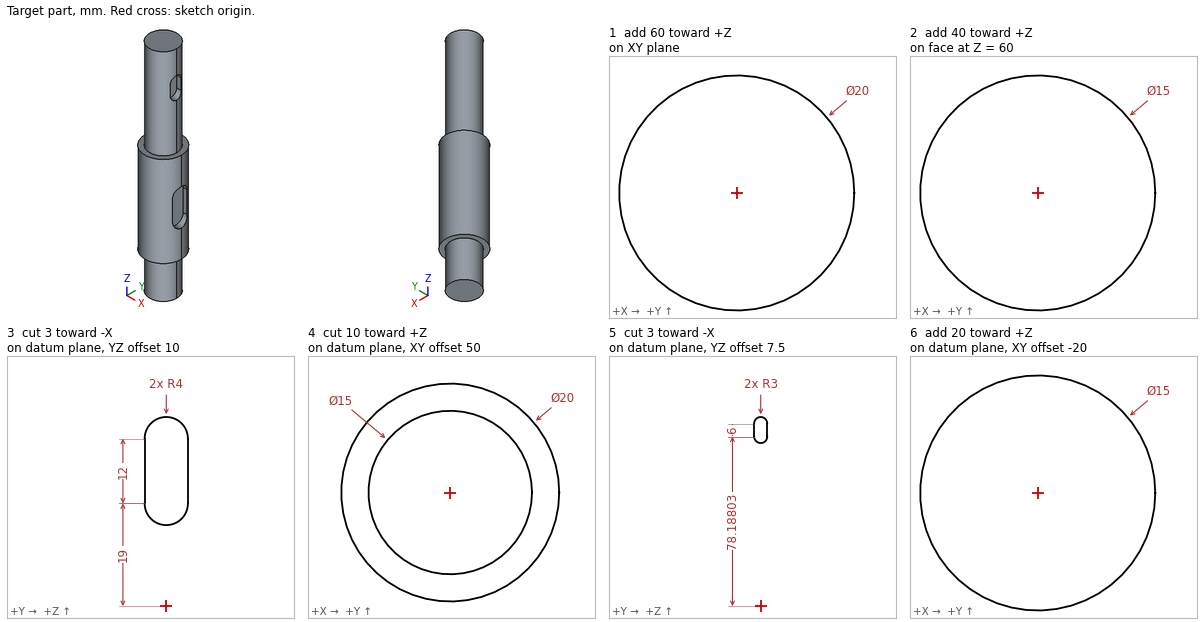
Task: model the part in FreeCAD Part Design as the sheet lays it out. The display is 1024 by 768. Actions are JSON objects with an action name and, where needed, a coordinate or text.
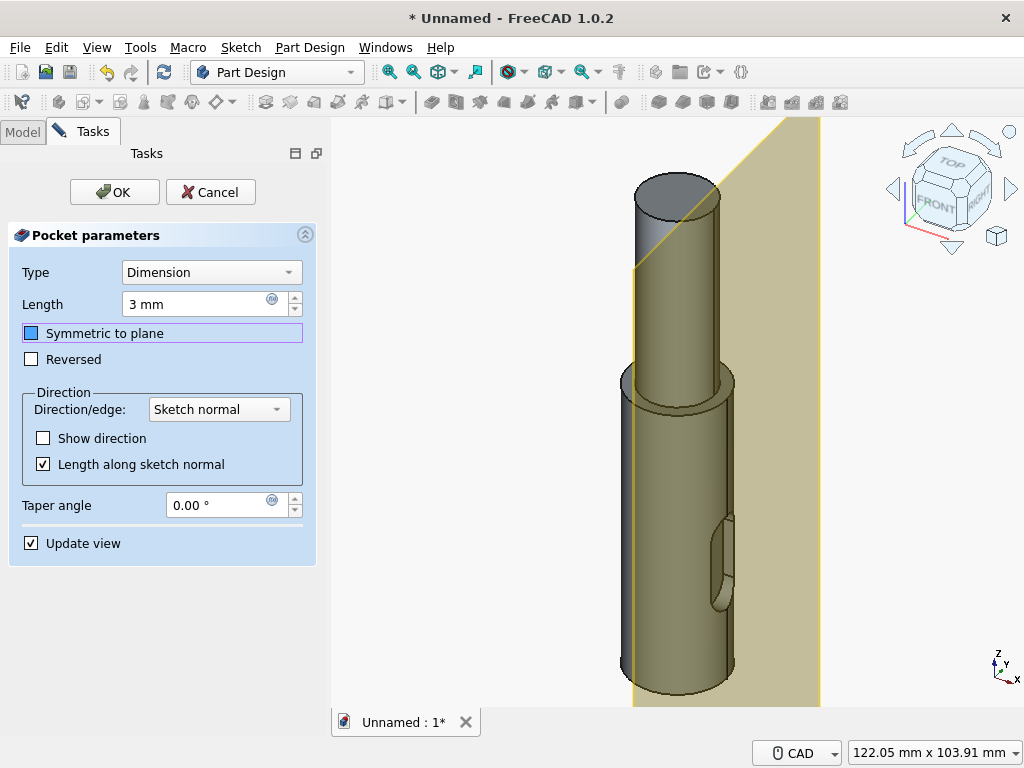
{"action": "left_click", "coordinate": [115, 192]}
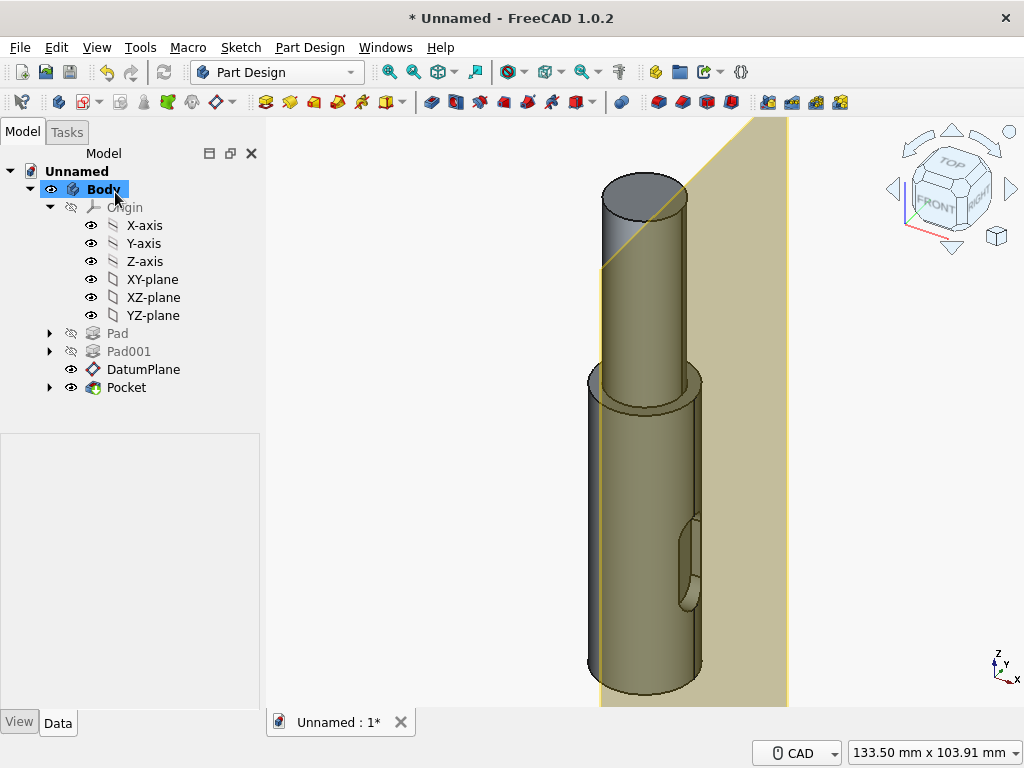
{"action": "left_click", "coordinate": [116, 369]}
{"action": "key", "text": "space"}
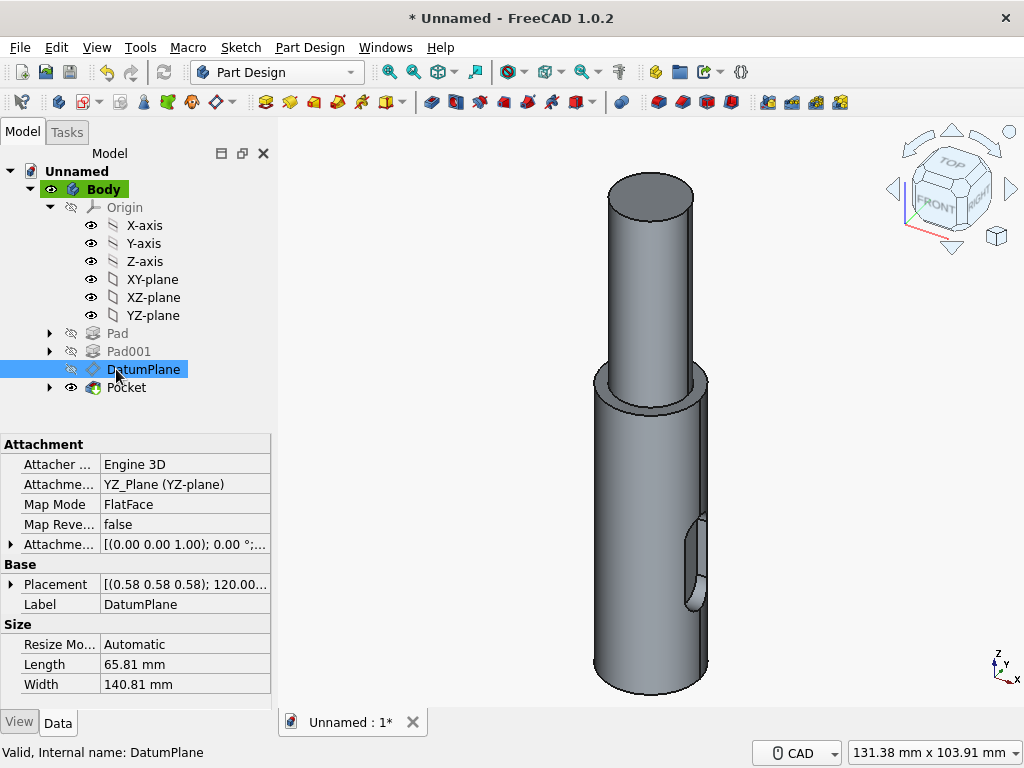
{"action": "left_click", "coordinate": [136, 279]}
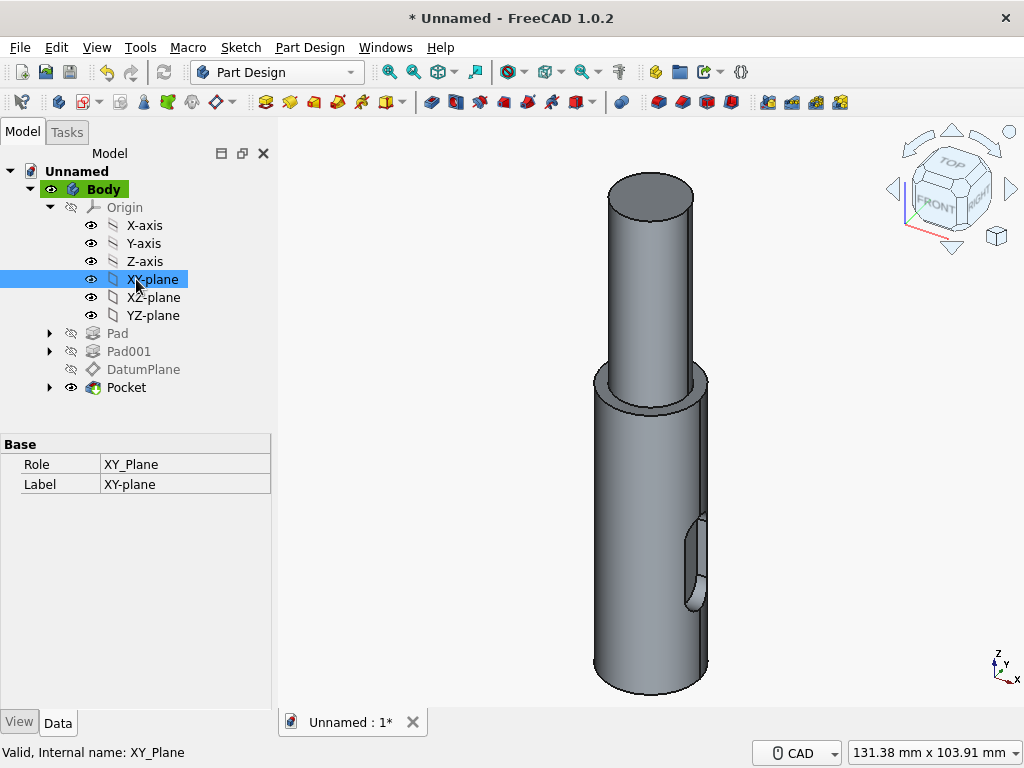
{"action": "left_click", "coordinate": [216, 102]}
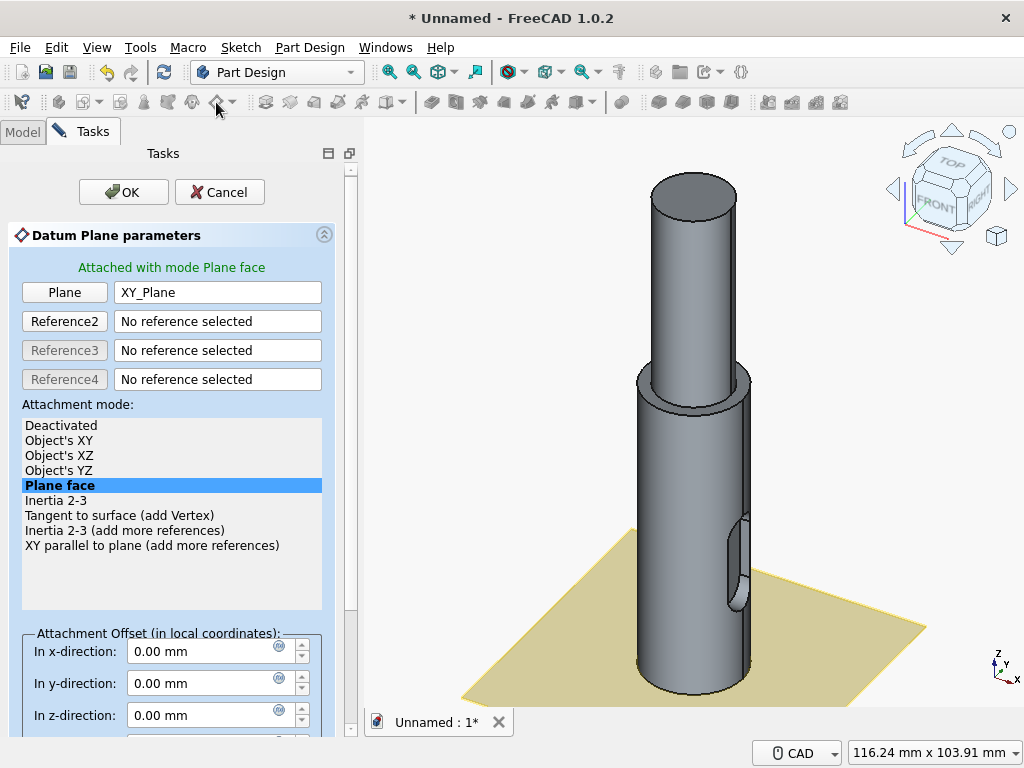
{"action": "triple_click", "coordinate": [210, 715]}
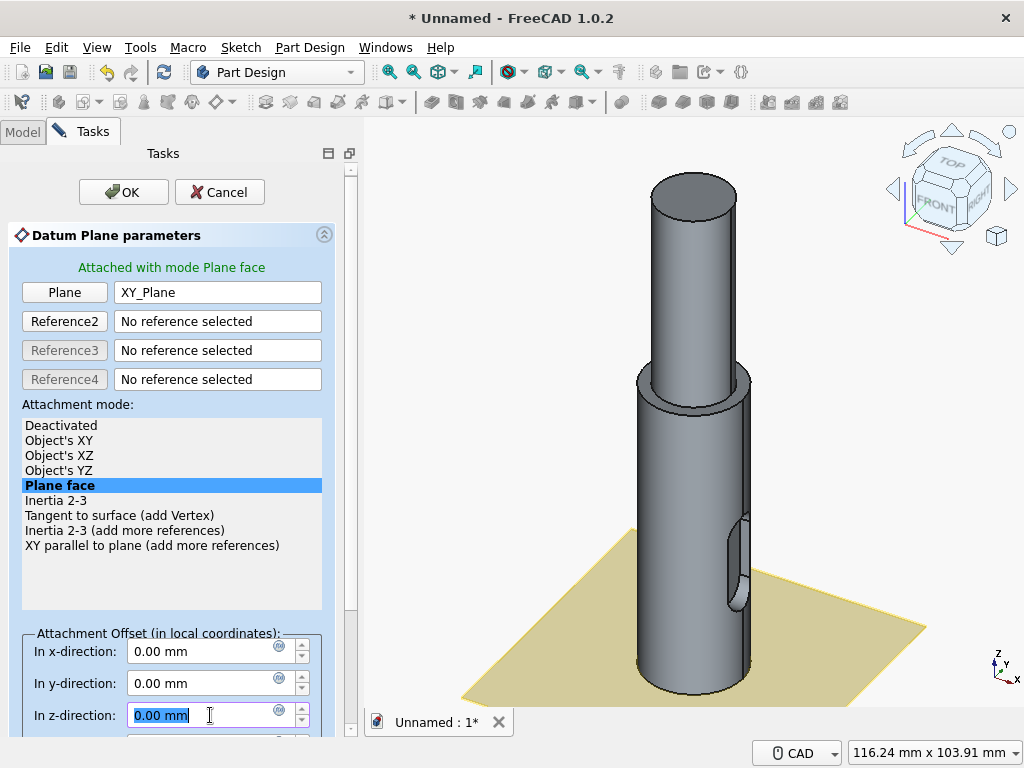
{"action": "type", "text": "50"}
{"action": "key", "text": "Tab"}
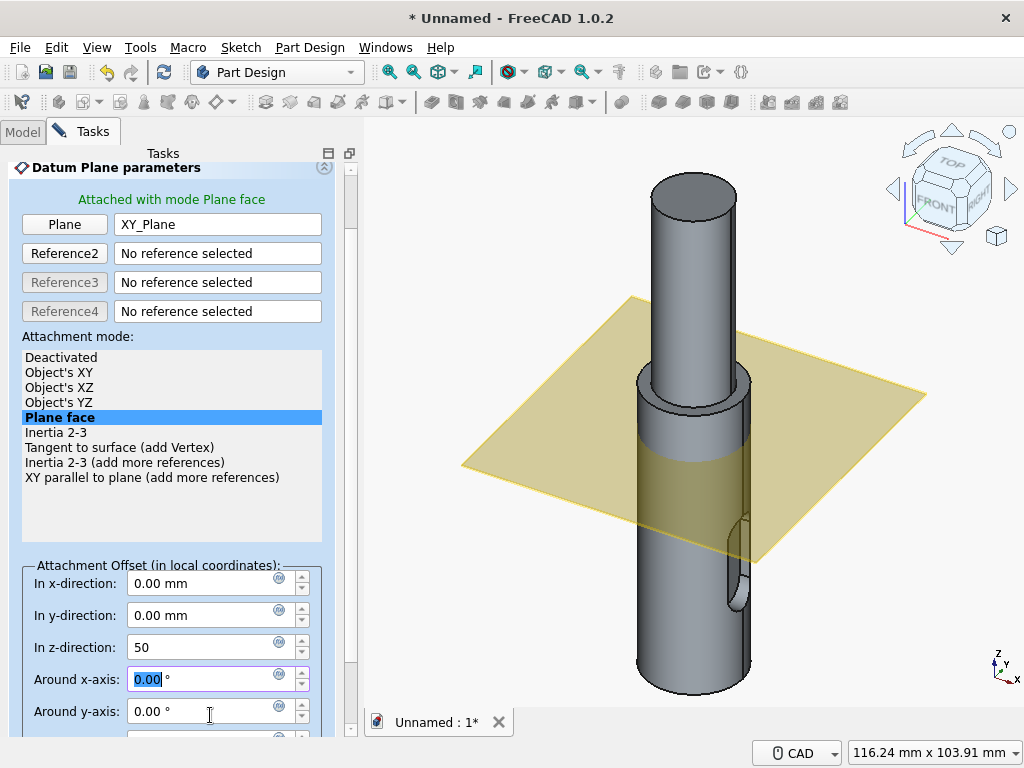
{"action": "scroll", "coordinate": [351, 450], "scroll_direction": "up", "scroll_amount": 2}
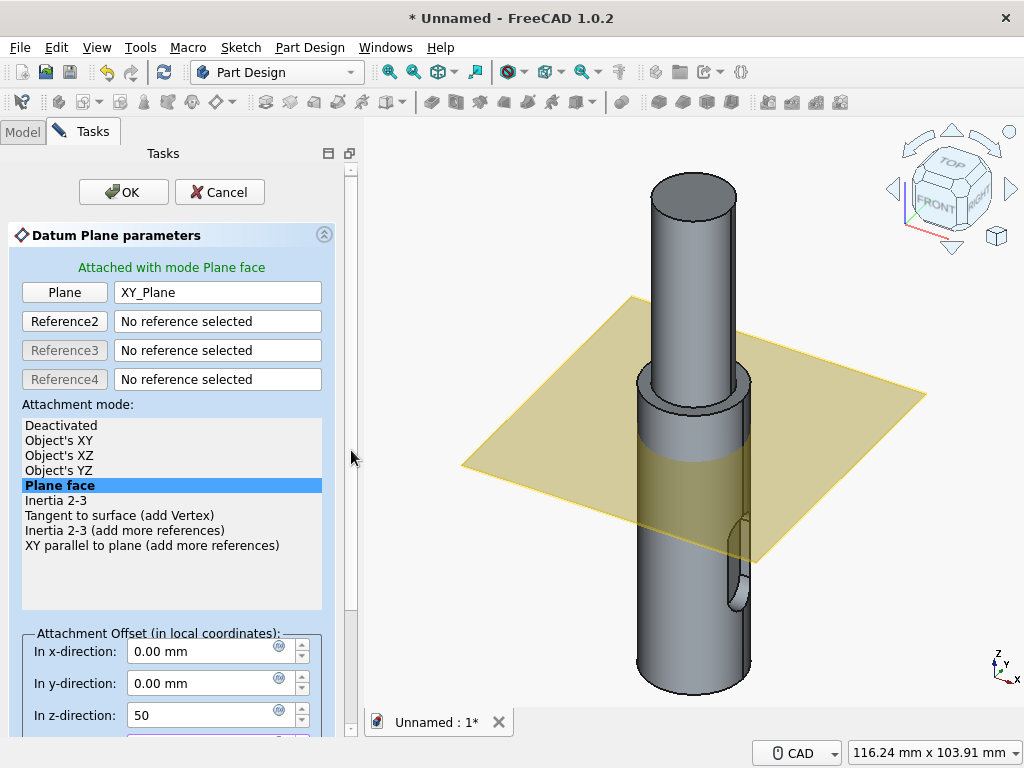
{"action": "left_click", "coordinate": [124, 192]}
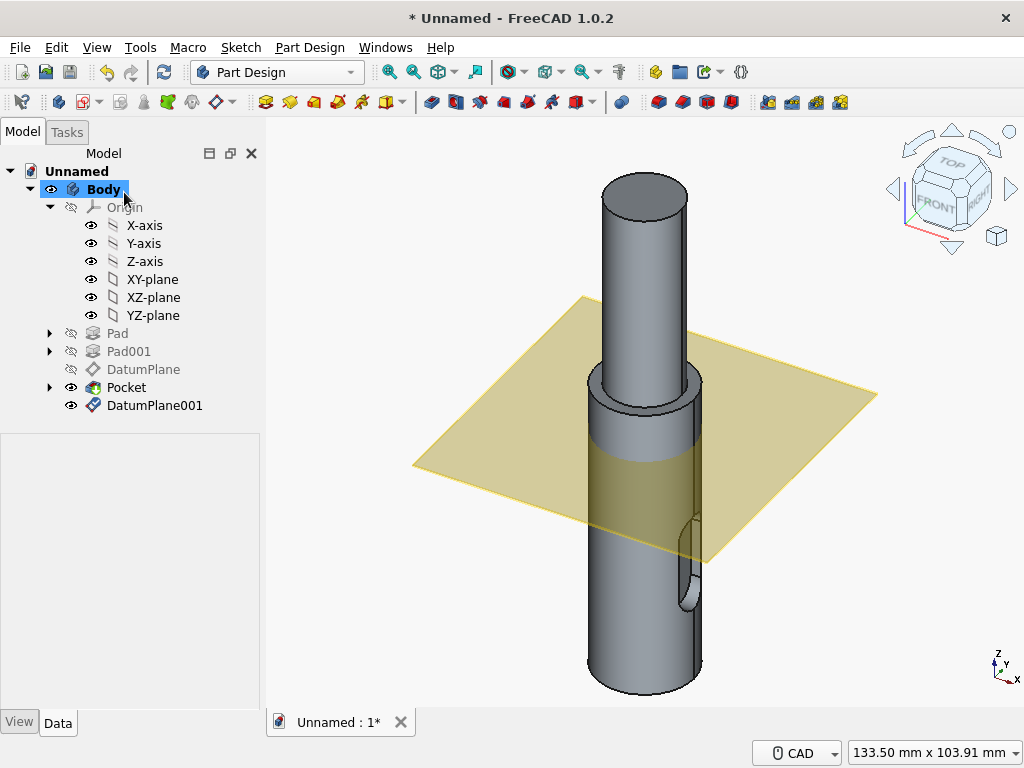
{"action": "left_click", "coordinate": [116, 405]}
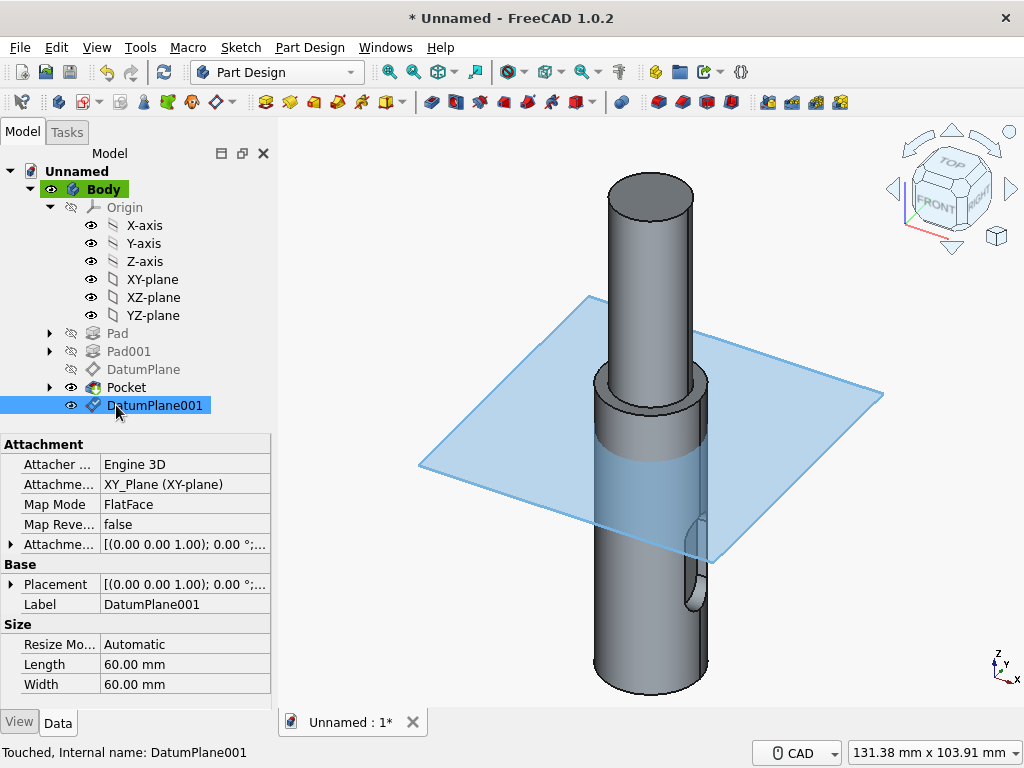
{"action": "left_click", "coordinate": [84, 102]}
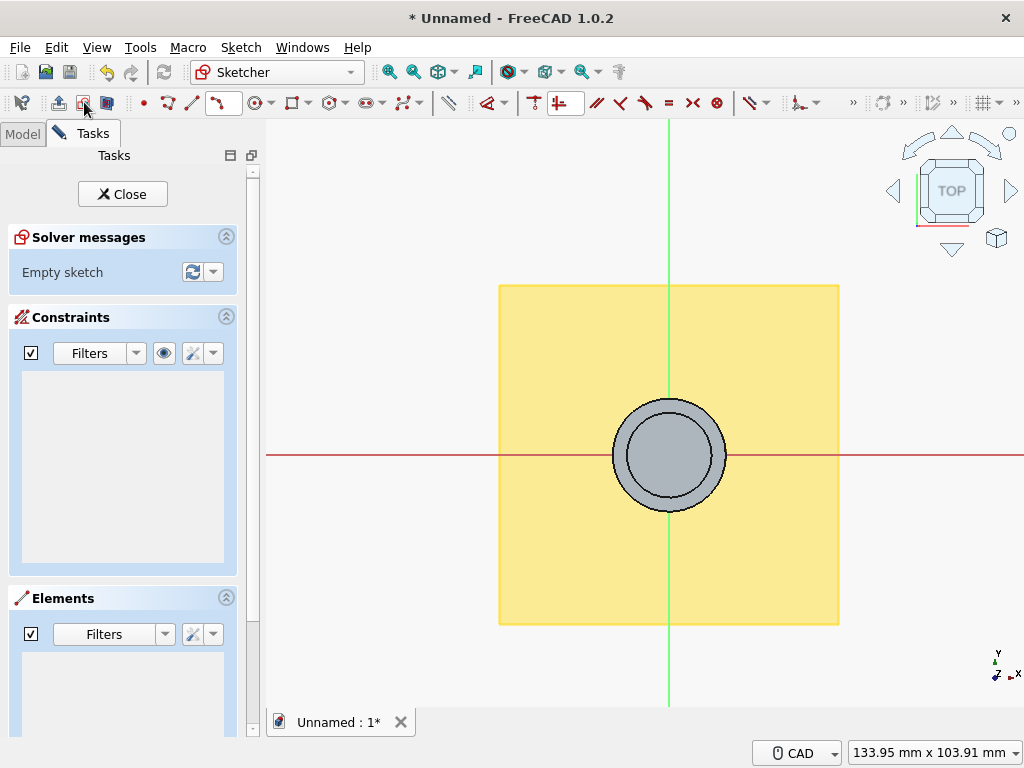
{"action": "left_click", "coordinate": [108, 104]}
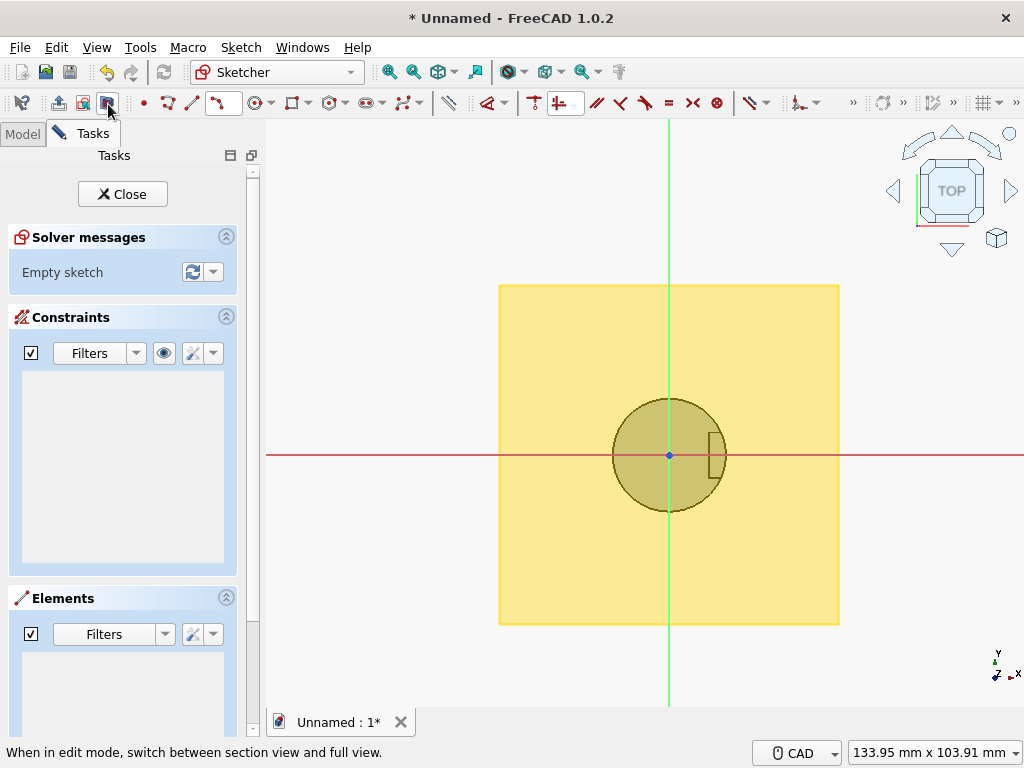
{"action": "scroll", "coordinate": [709, 473], "scroll_direction": "up", "scroll_amount": 6}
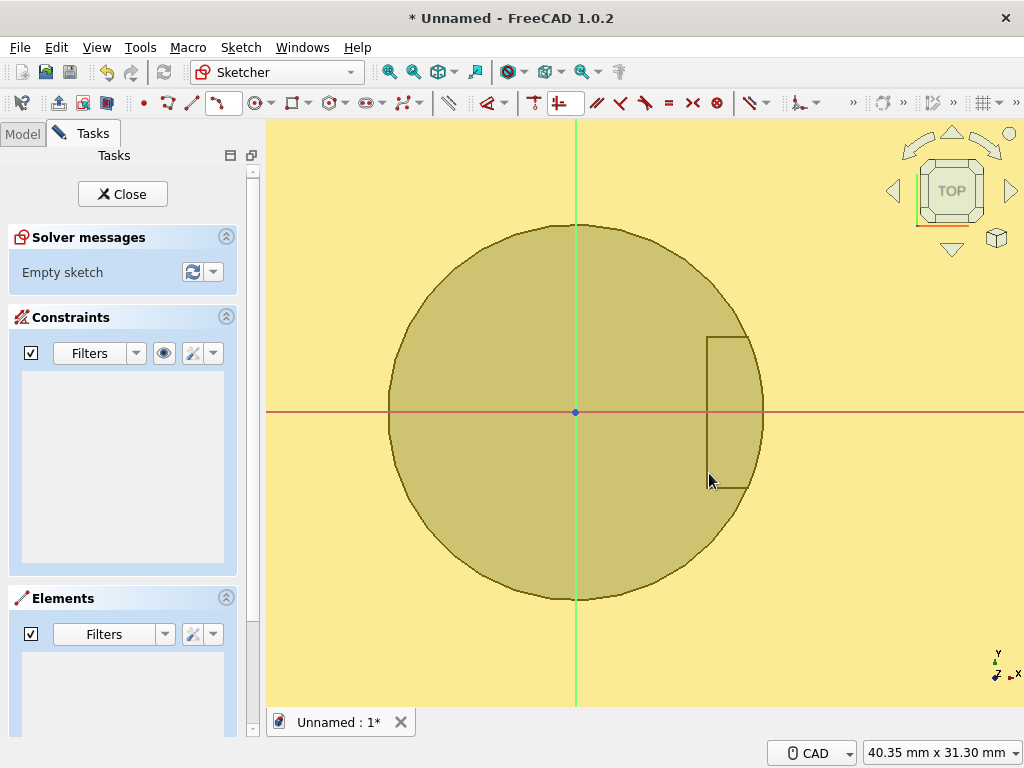
{"action": "left_click", "coordinate": [256, 104]}